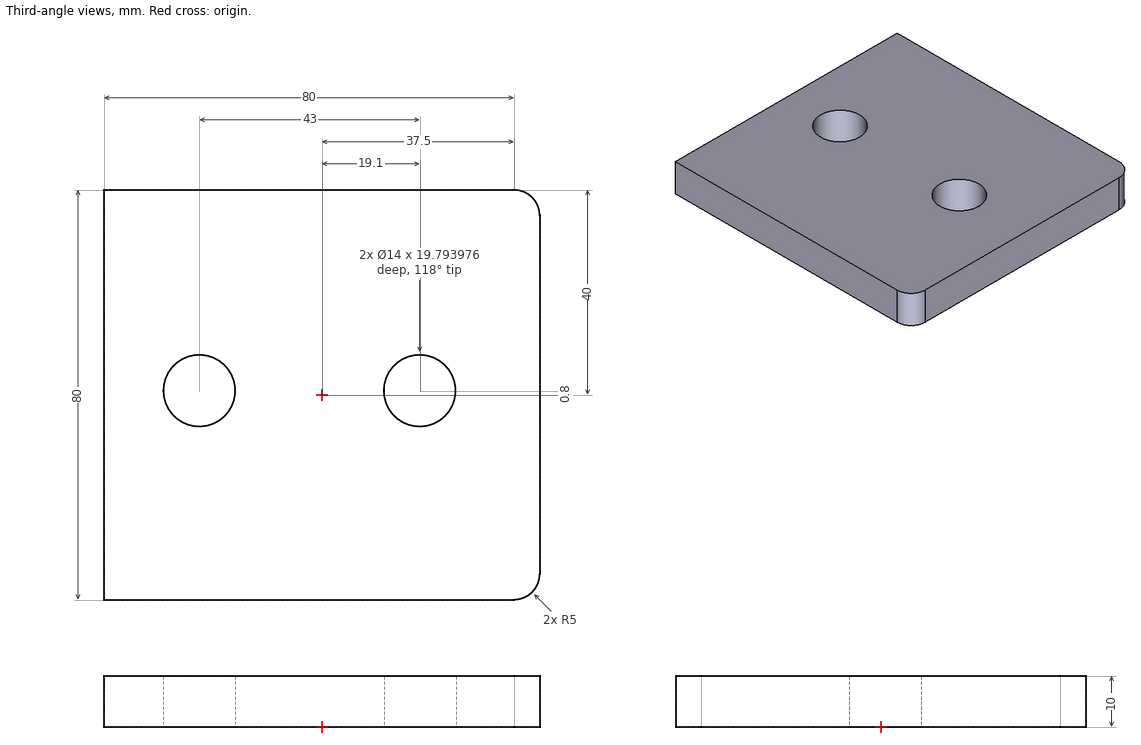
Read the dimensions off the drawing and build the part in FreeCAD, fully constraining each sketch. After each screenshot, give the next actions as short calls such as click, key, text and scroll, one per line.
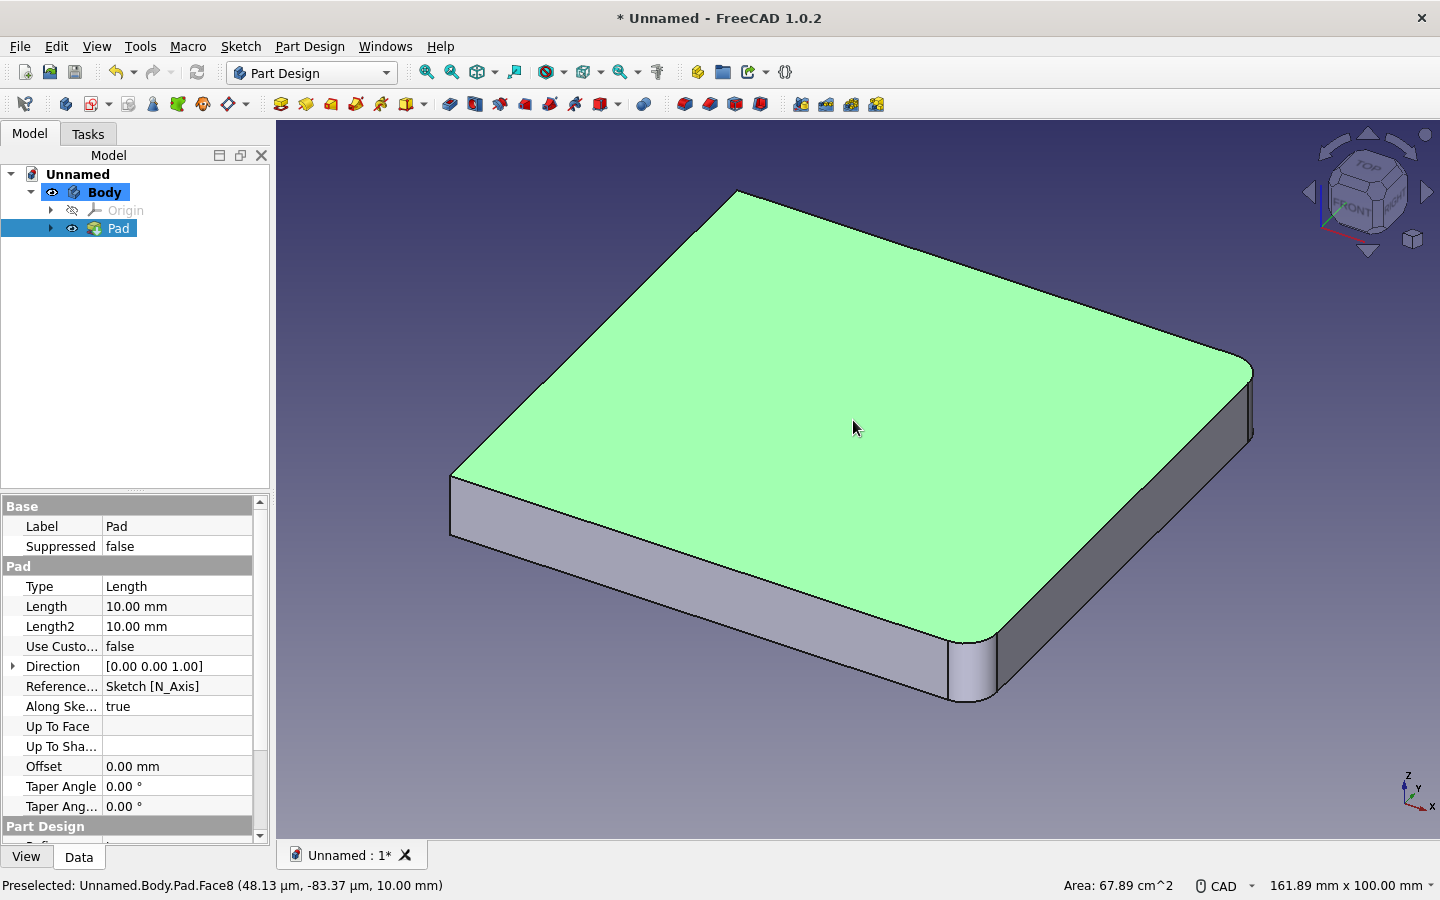
click(90, 104)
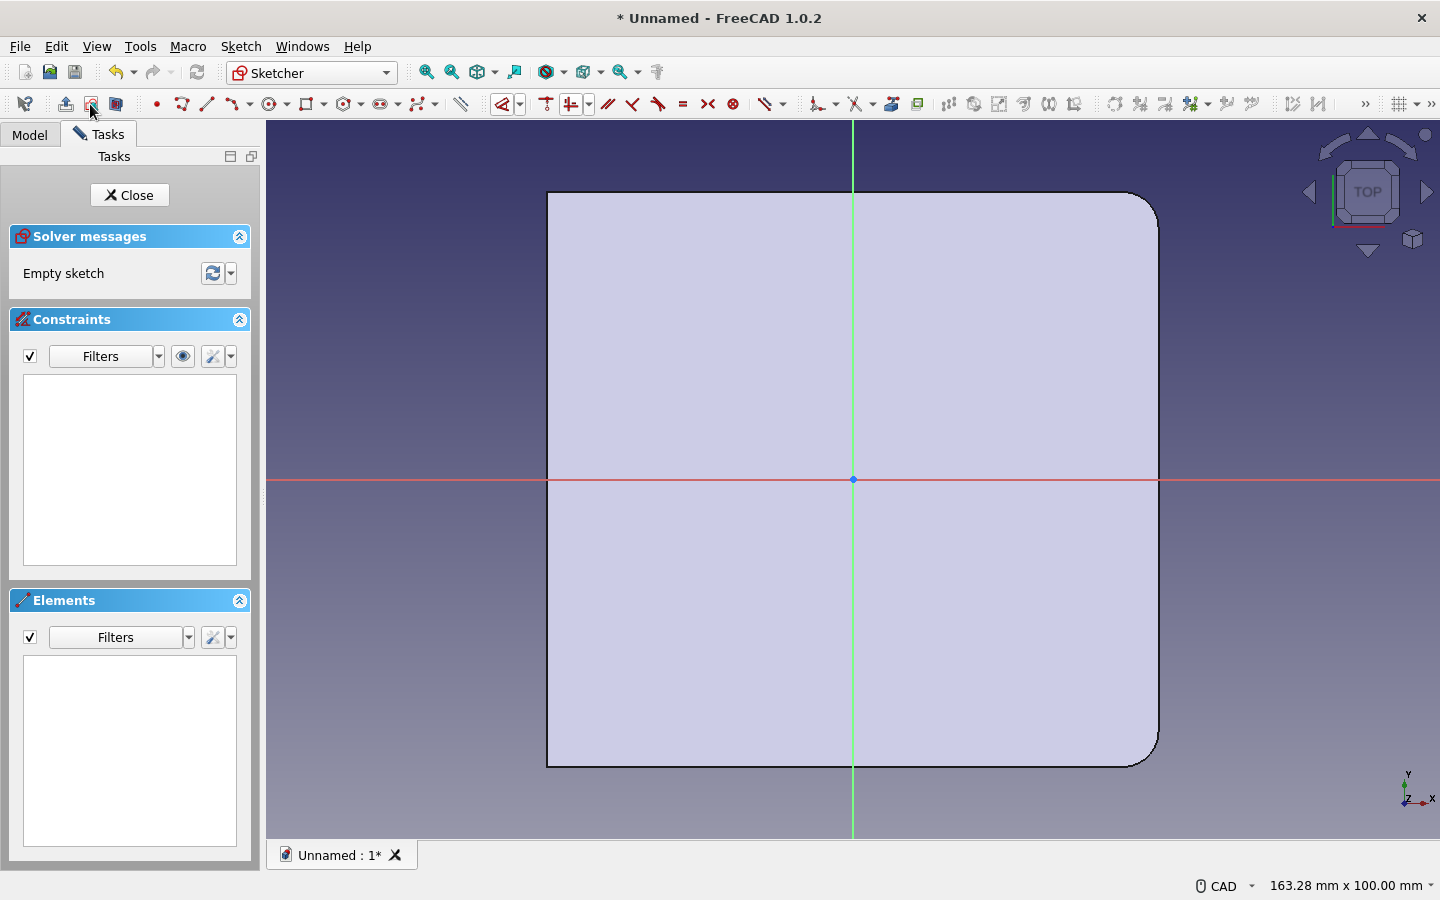
scroll(898, 467, up, 3)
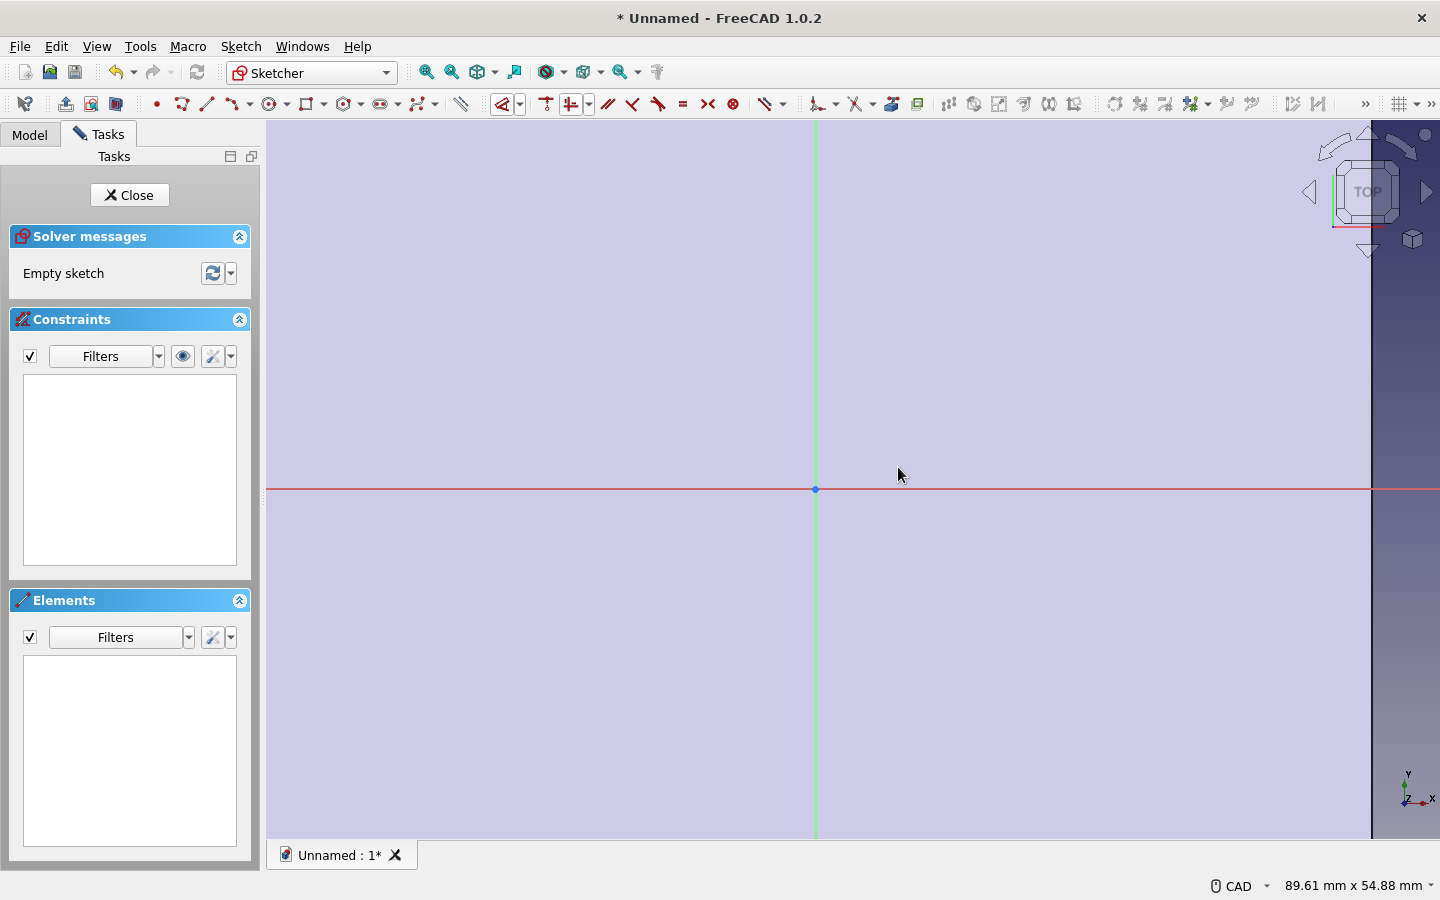
click(268, 104)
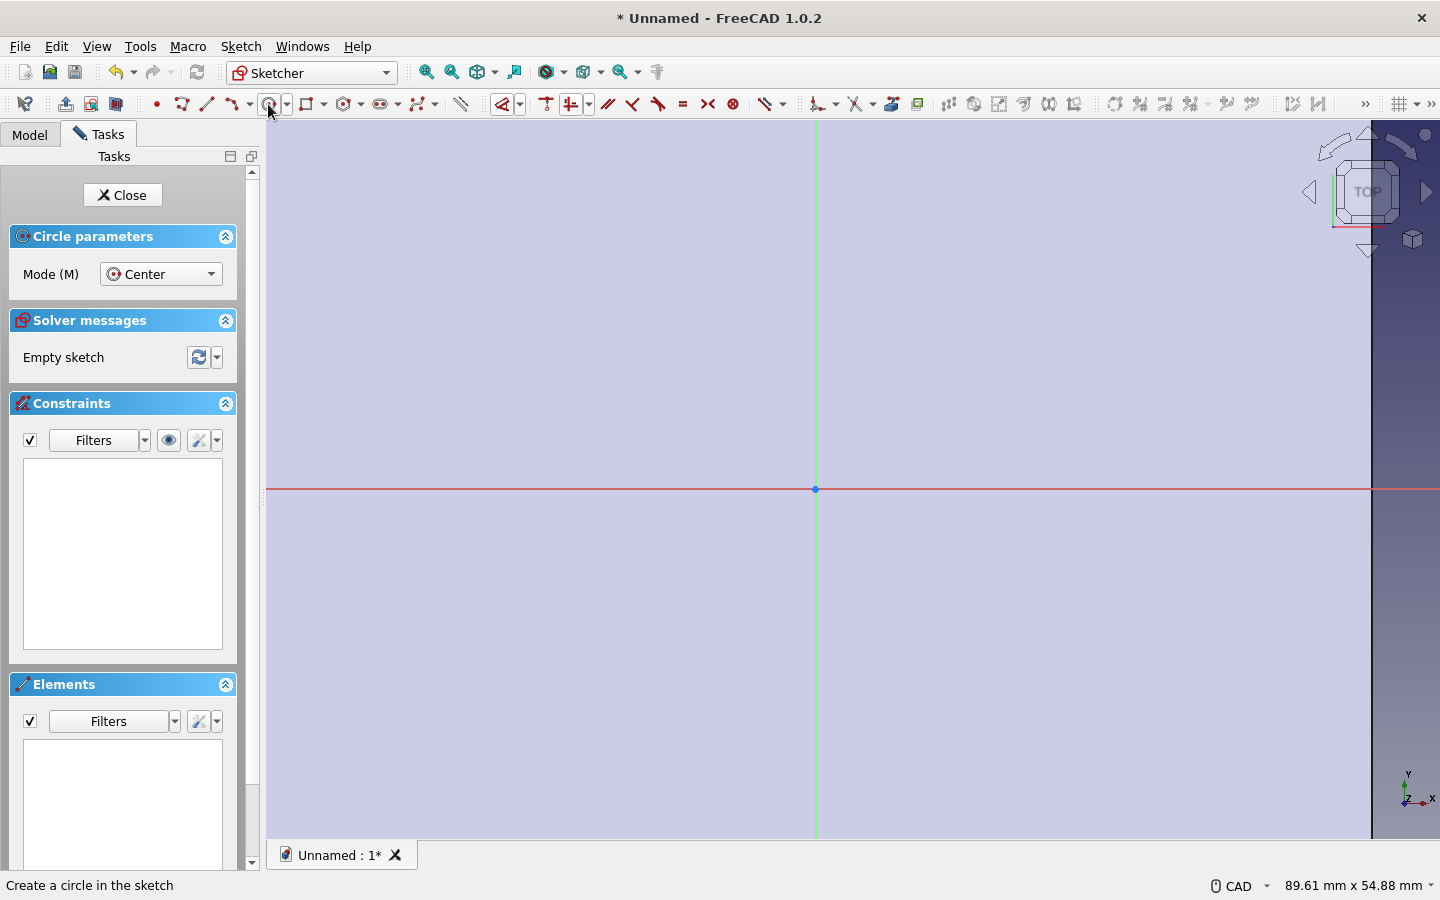
scroll(1066, 479, up, 3)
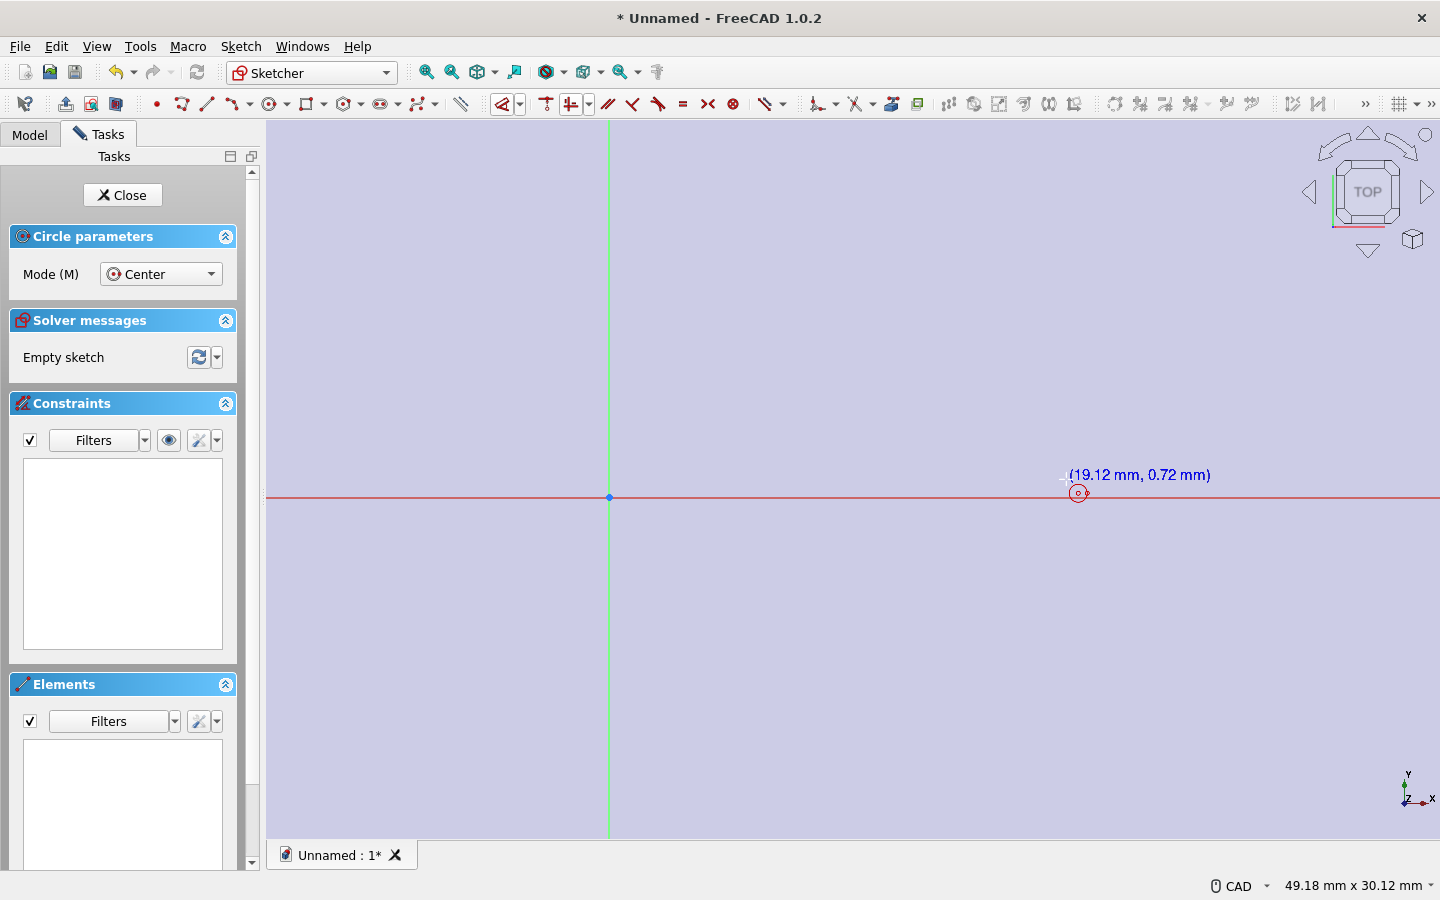
click(1065, 478)
click(1183, 360)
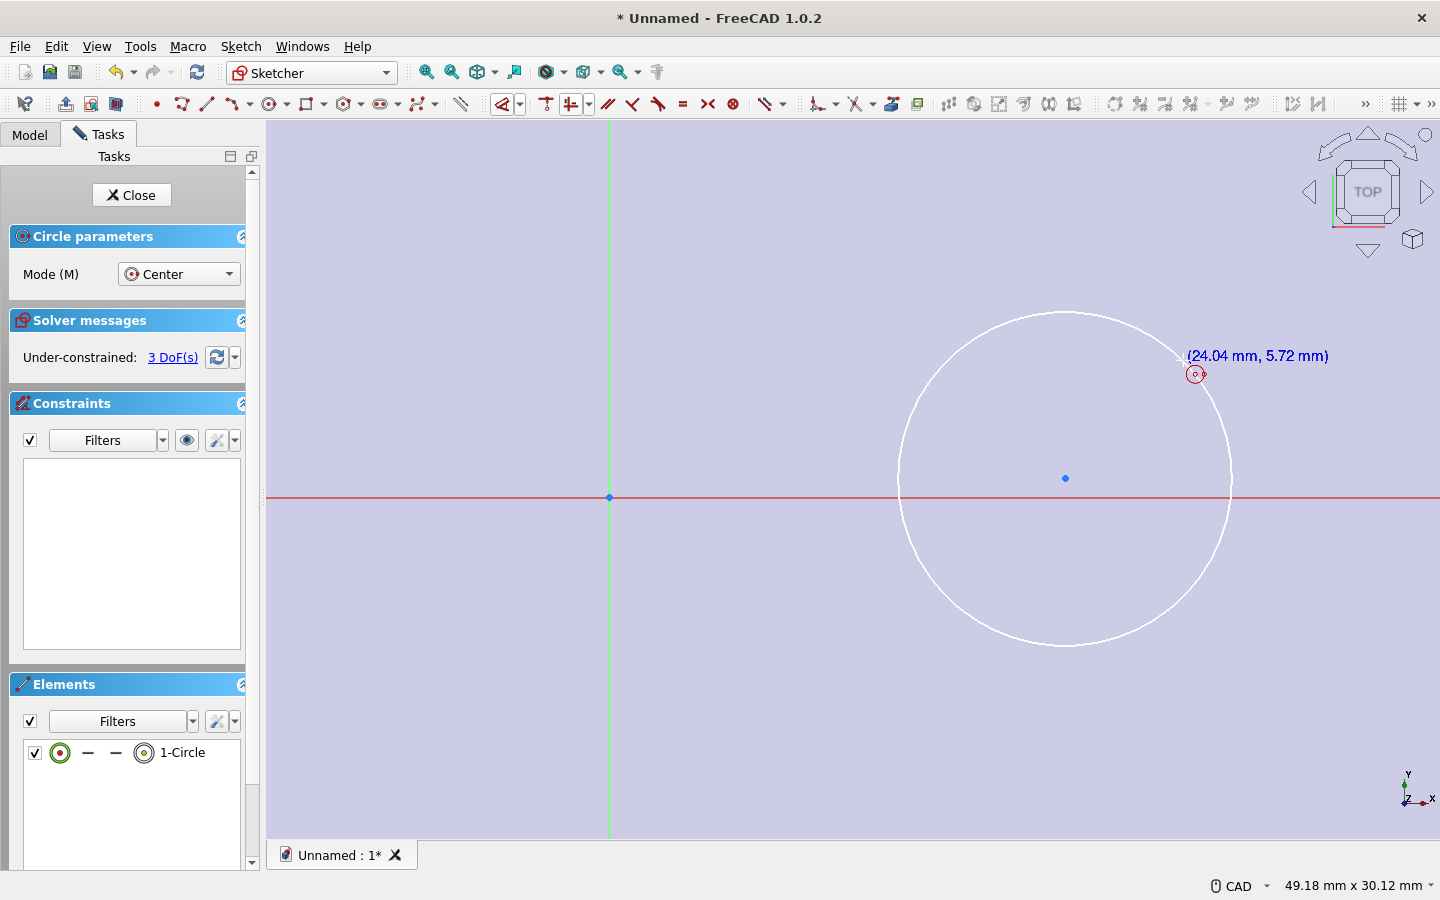
scroll(1068, 481, down, 3)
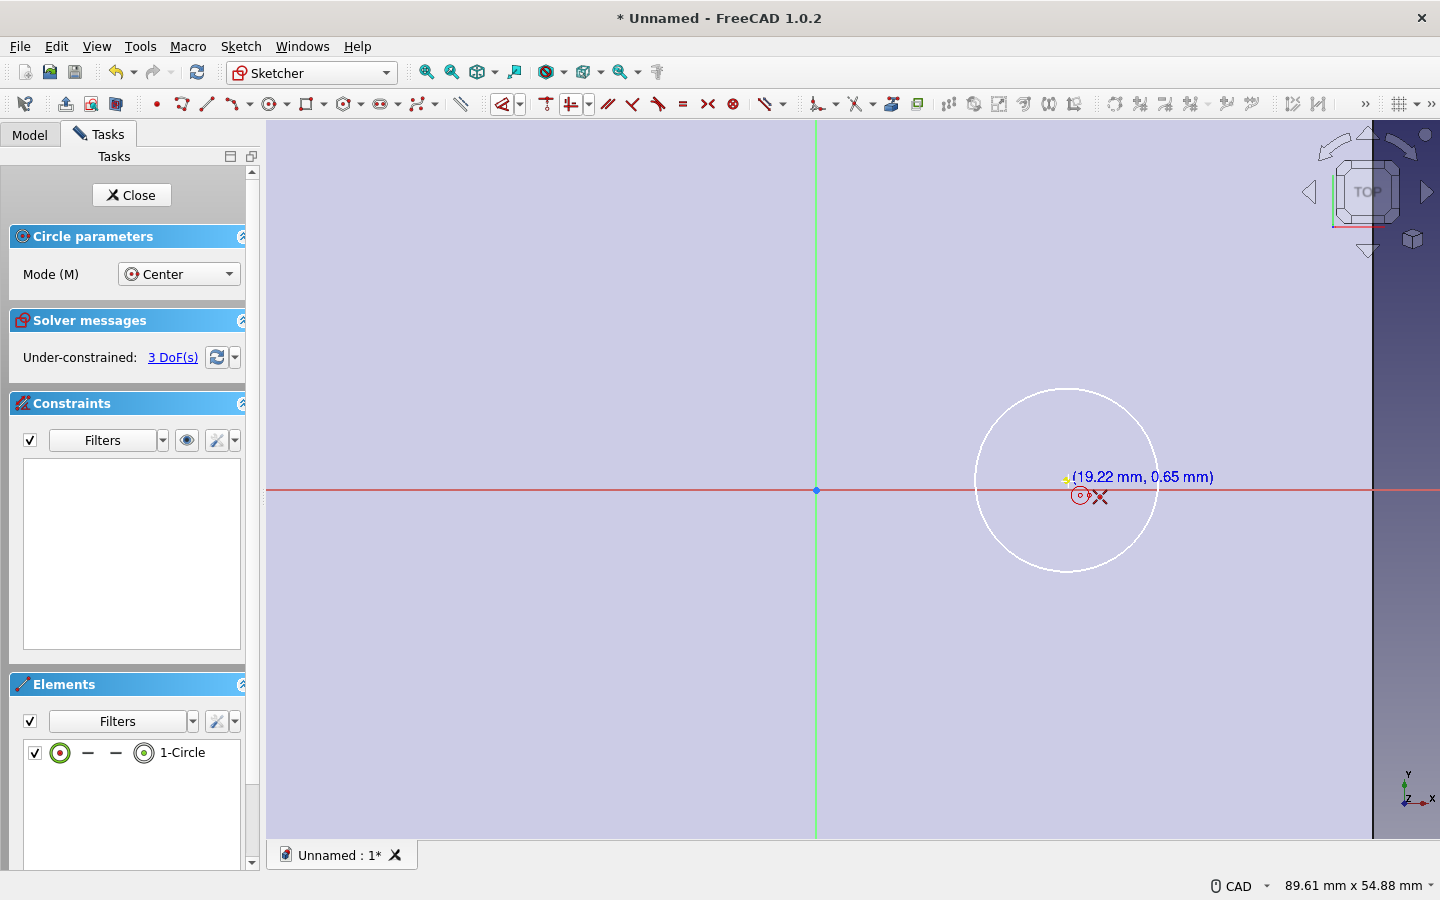
scroll(503, 480, up, 3)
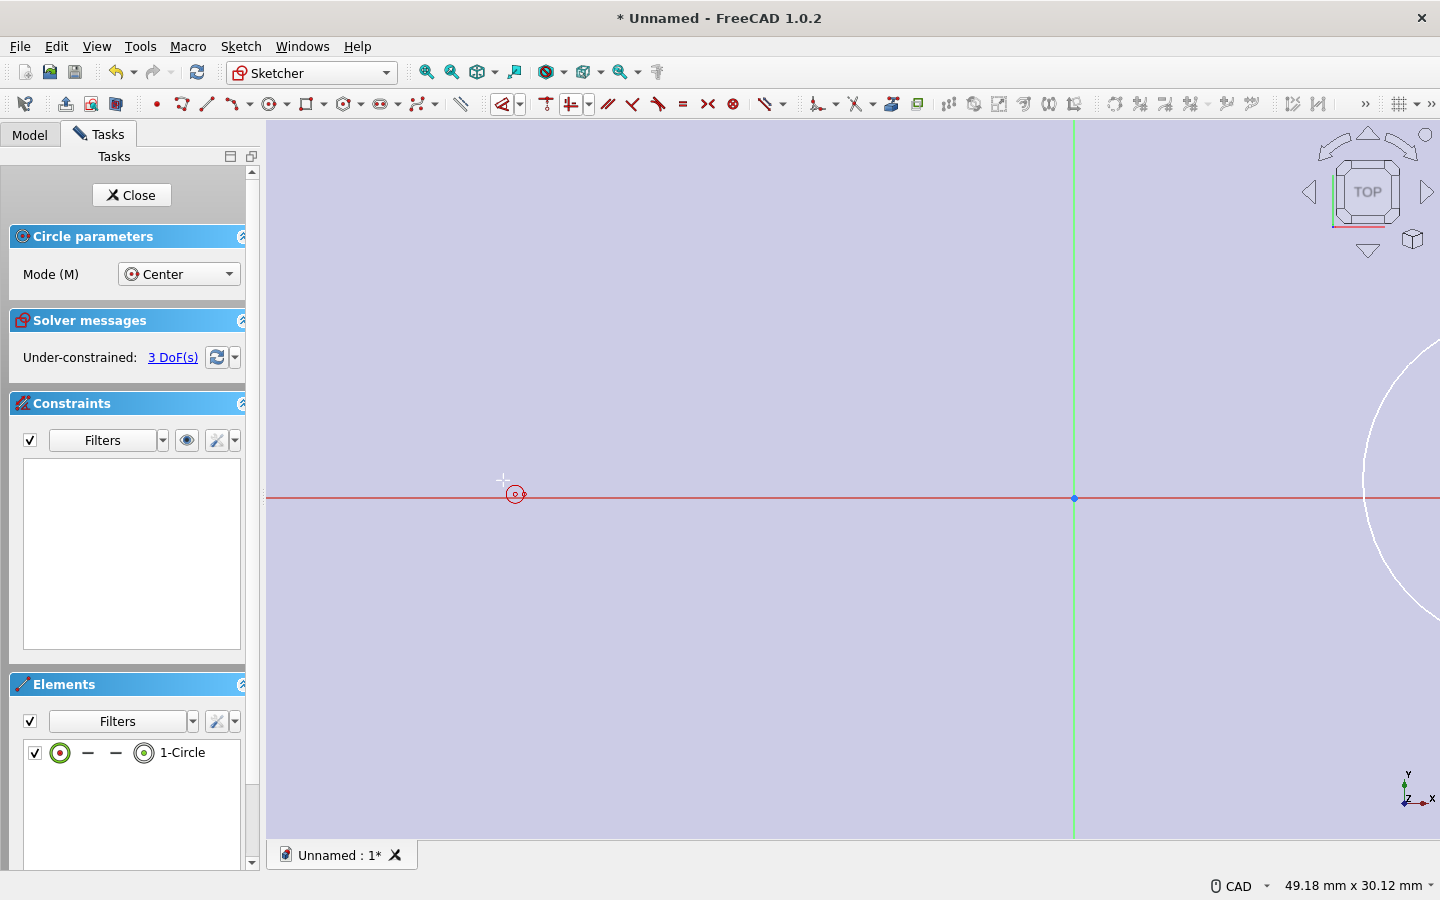
click(503, 479)
click(622, 361)
key(Escape)